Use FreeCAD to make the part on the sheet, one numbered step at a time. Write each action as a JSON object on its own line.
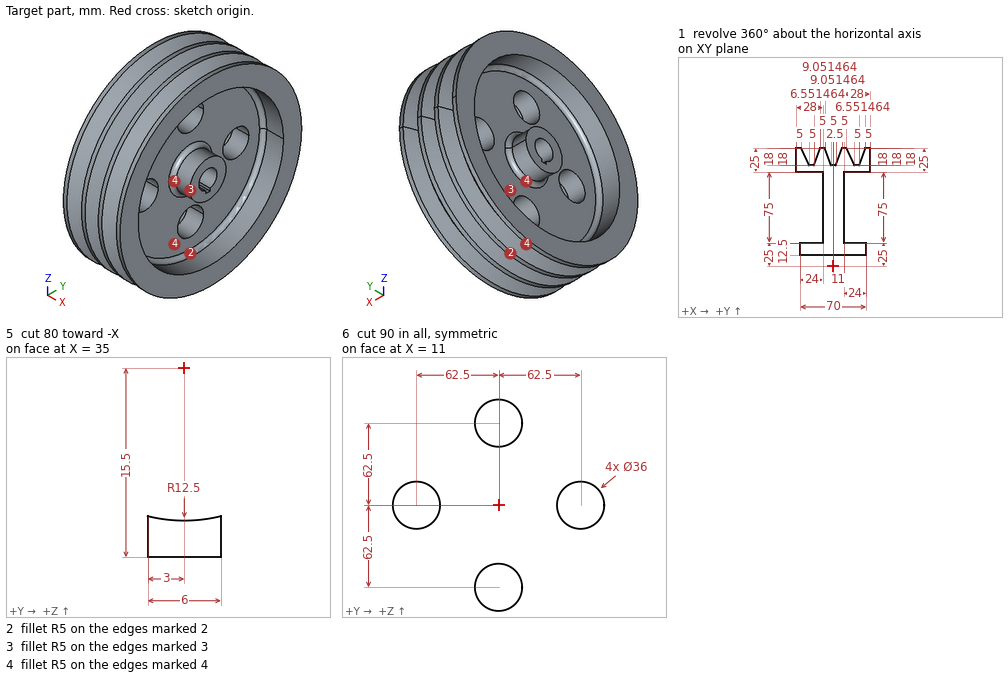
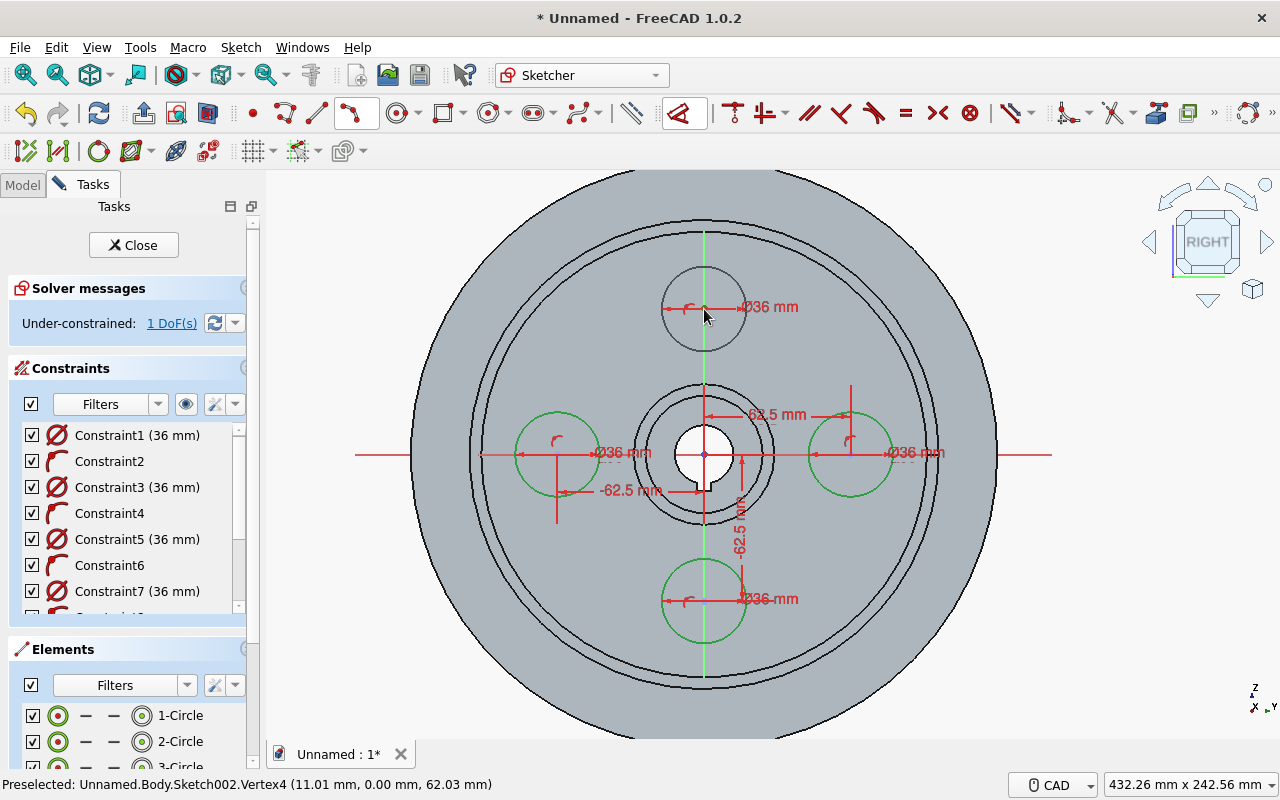
{"action": "left_click", "coordinate": [702, 114]}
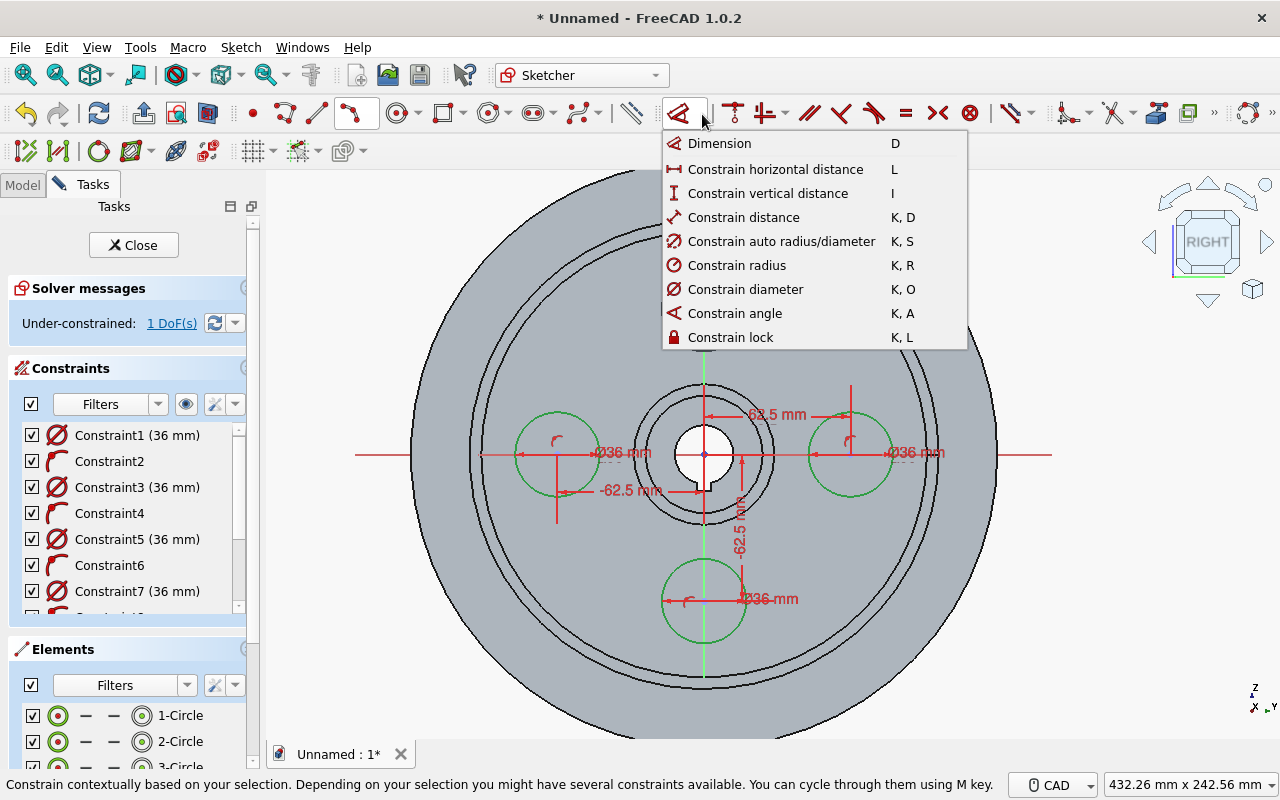
{"action": "left_click", "coordinate": [815, 193]}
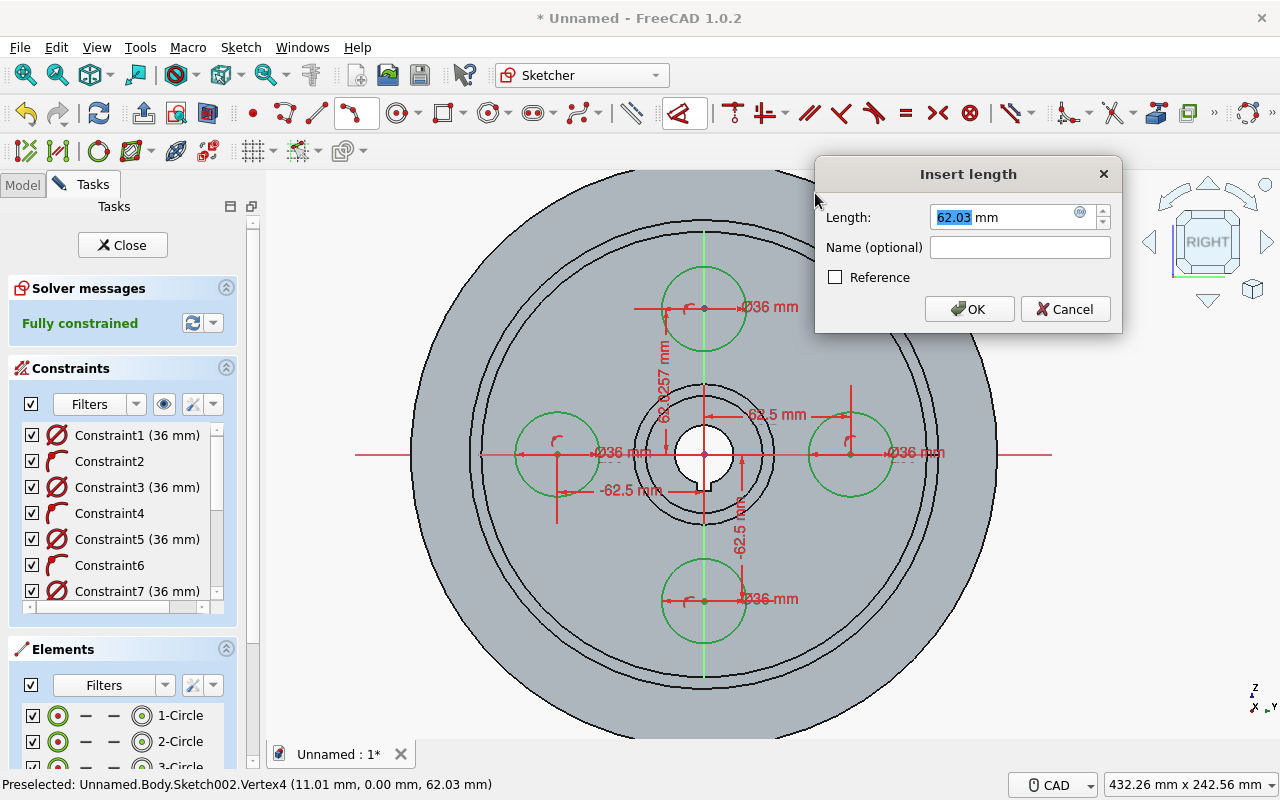
{"action": "type", "text": "62.5"}
{"action": "key", "text": "Return"}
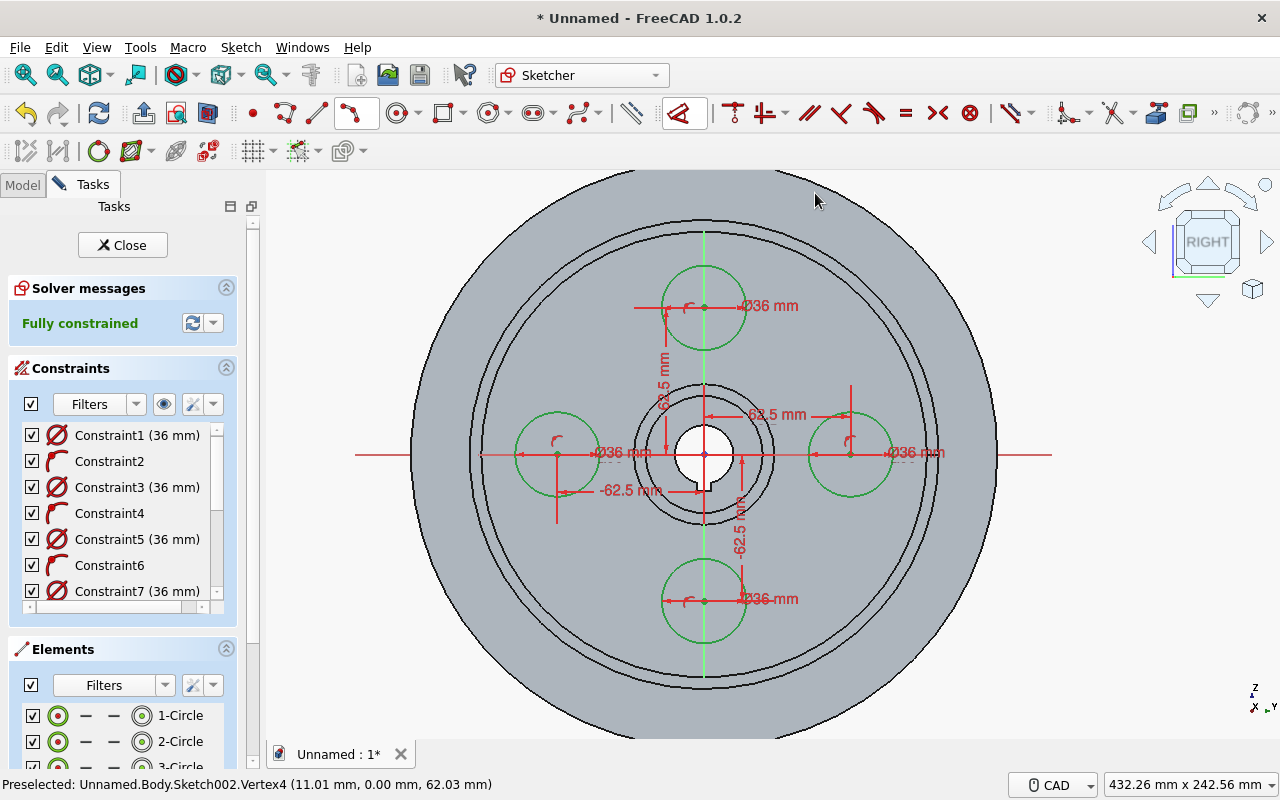
{"action": "left_click", "coordinate": [123, 245]}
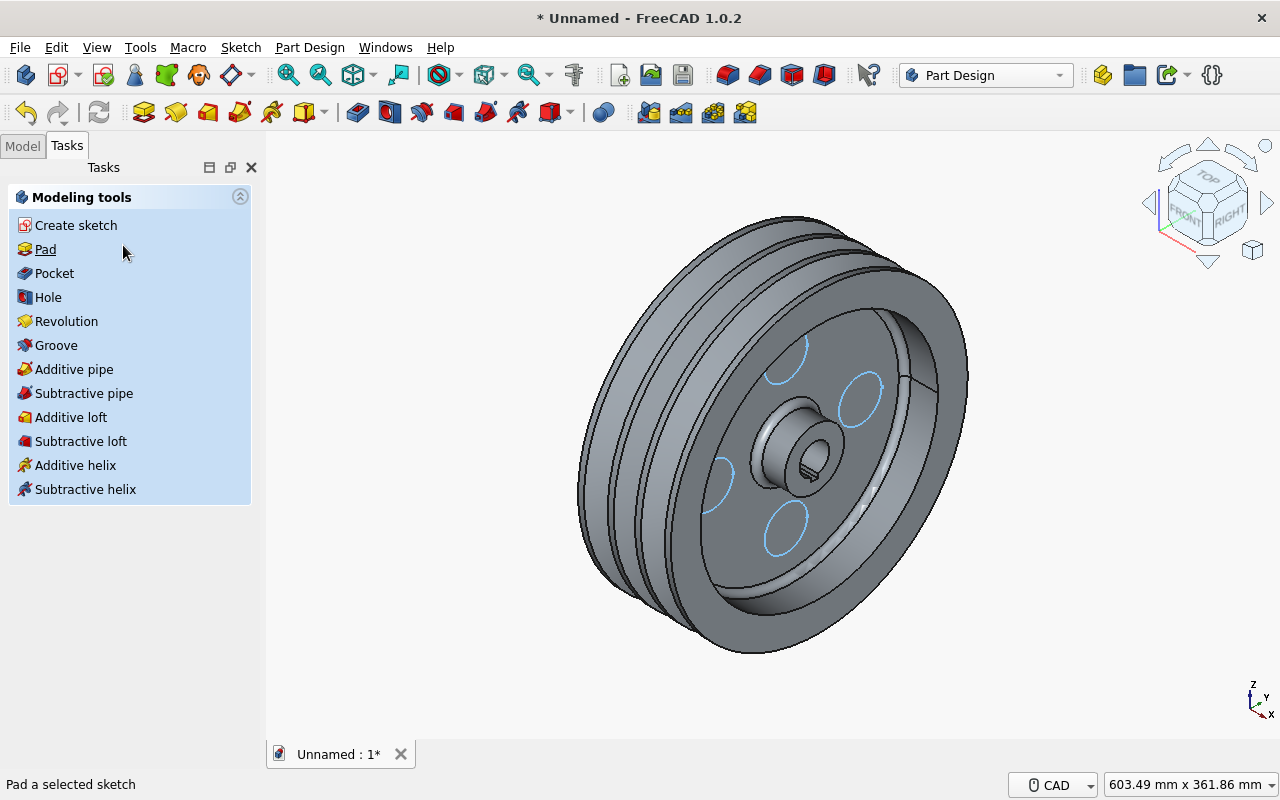
{"action": "left_click", "coordinate": [358, 112]}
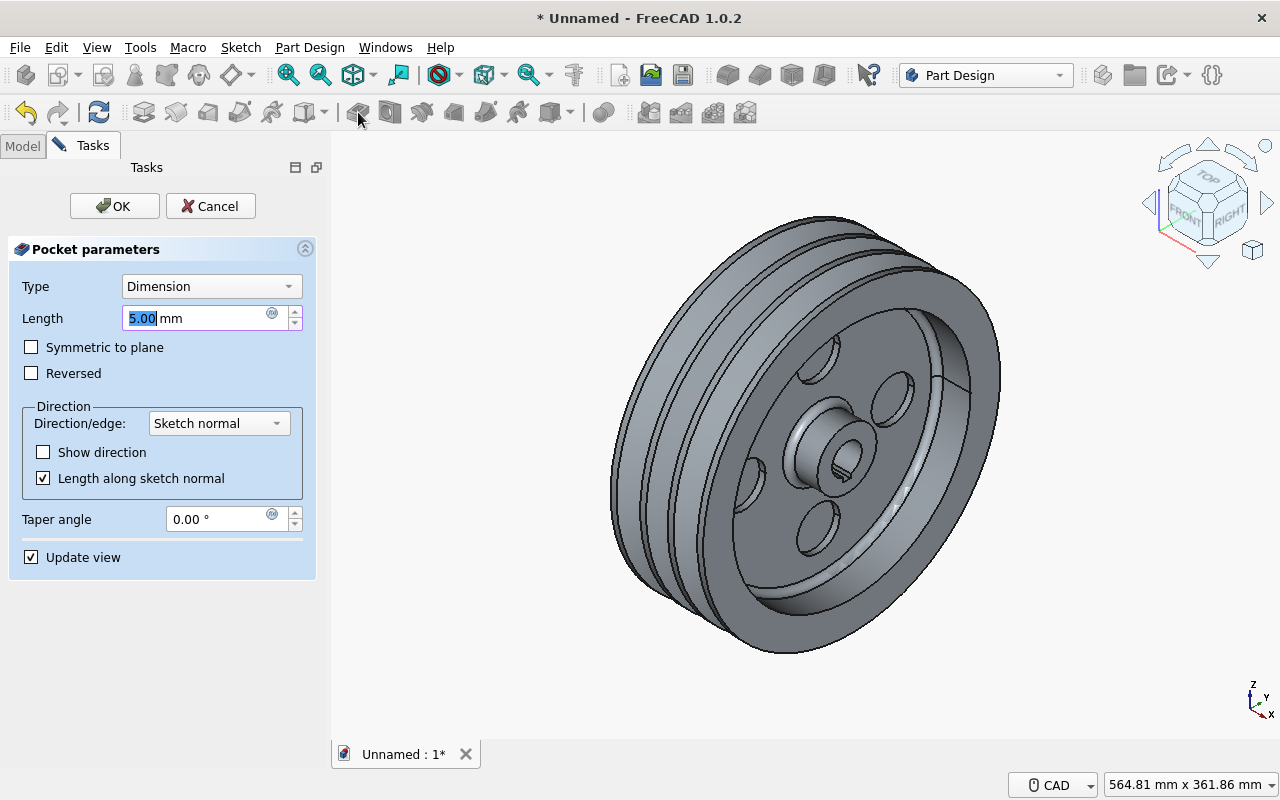
{"action": "type", "text": "90"}
{"action": "key", "text": "Tab"}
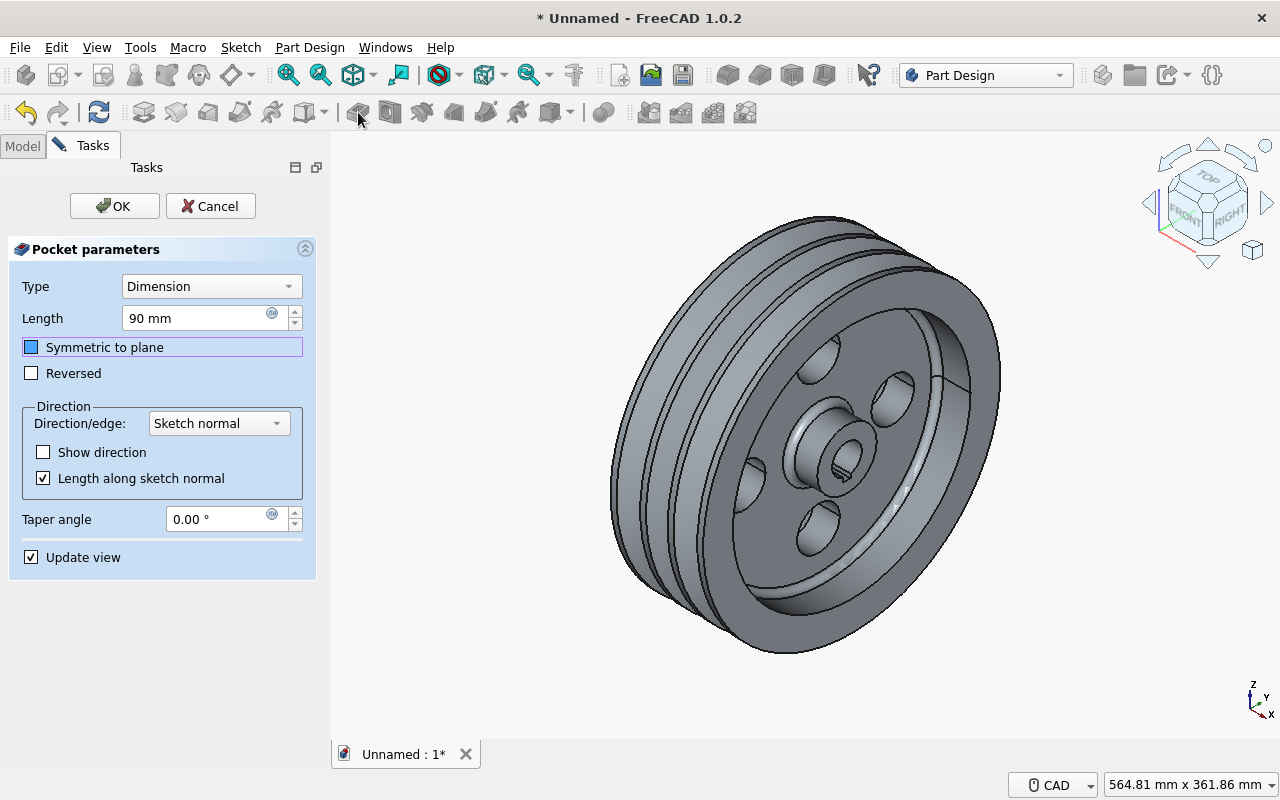
{"action": "left_click", "coordinate": [30, 347]}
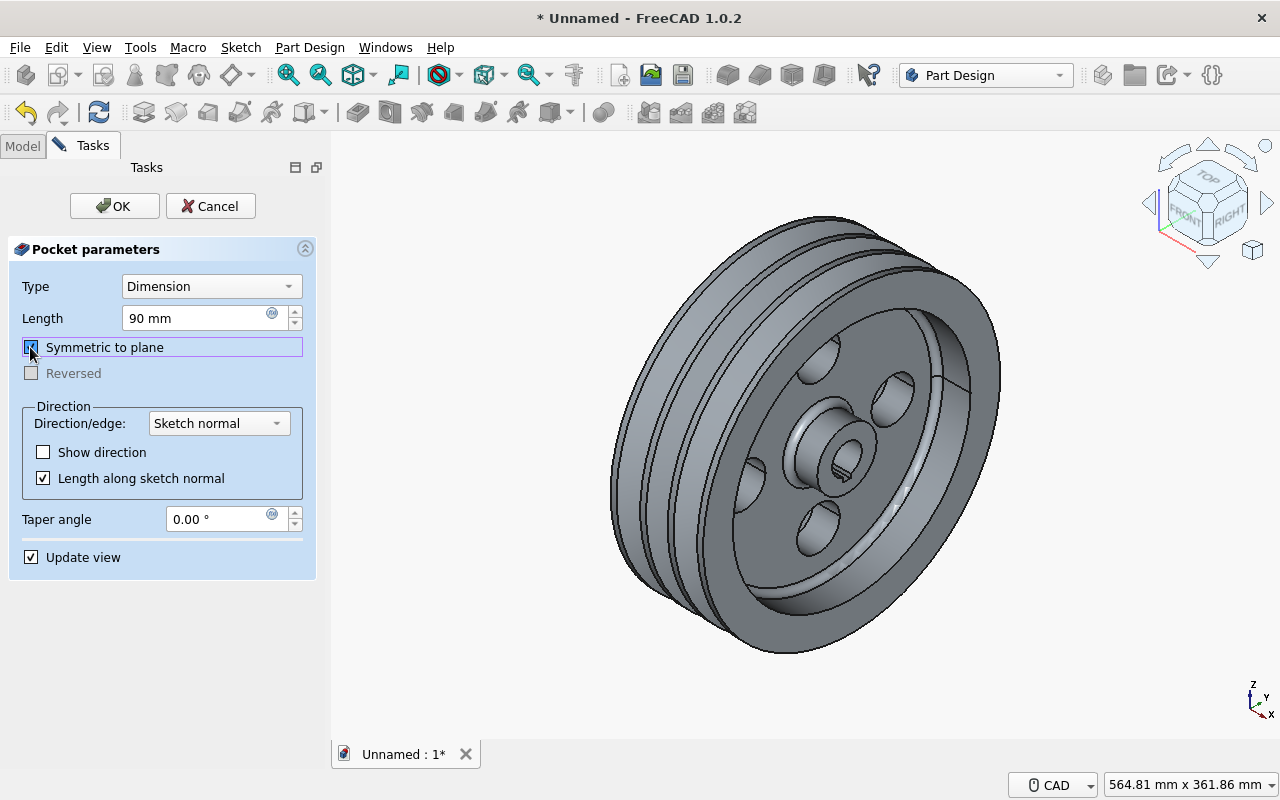
{"action": "left_click", "coordinate": [115, 206]}